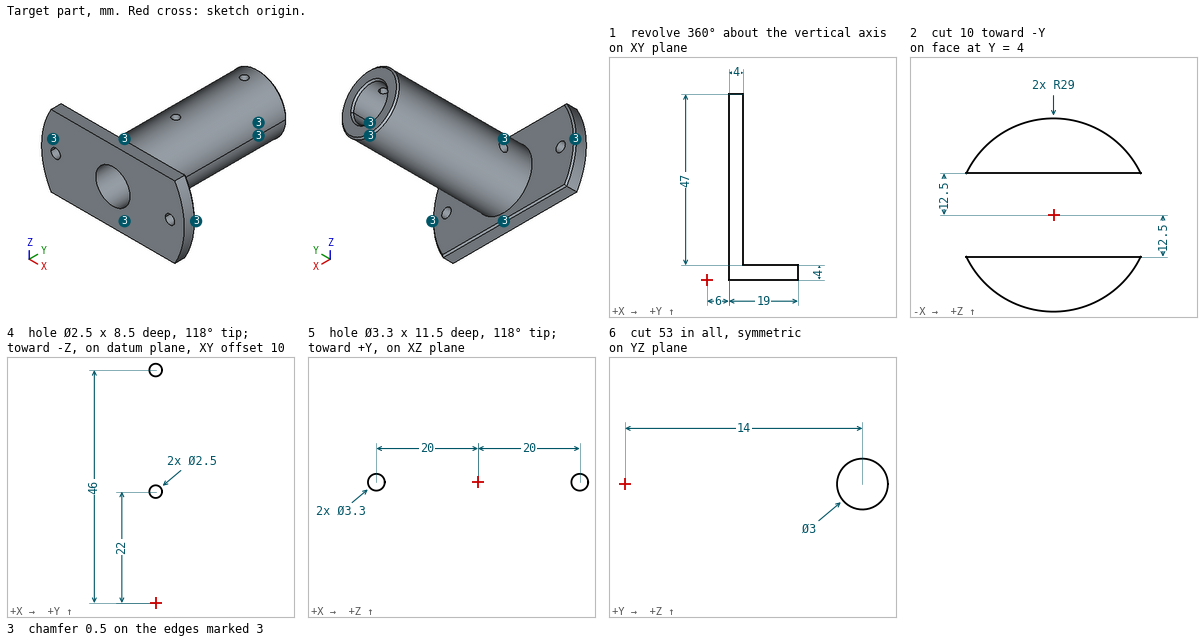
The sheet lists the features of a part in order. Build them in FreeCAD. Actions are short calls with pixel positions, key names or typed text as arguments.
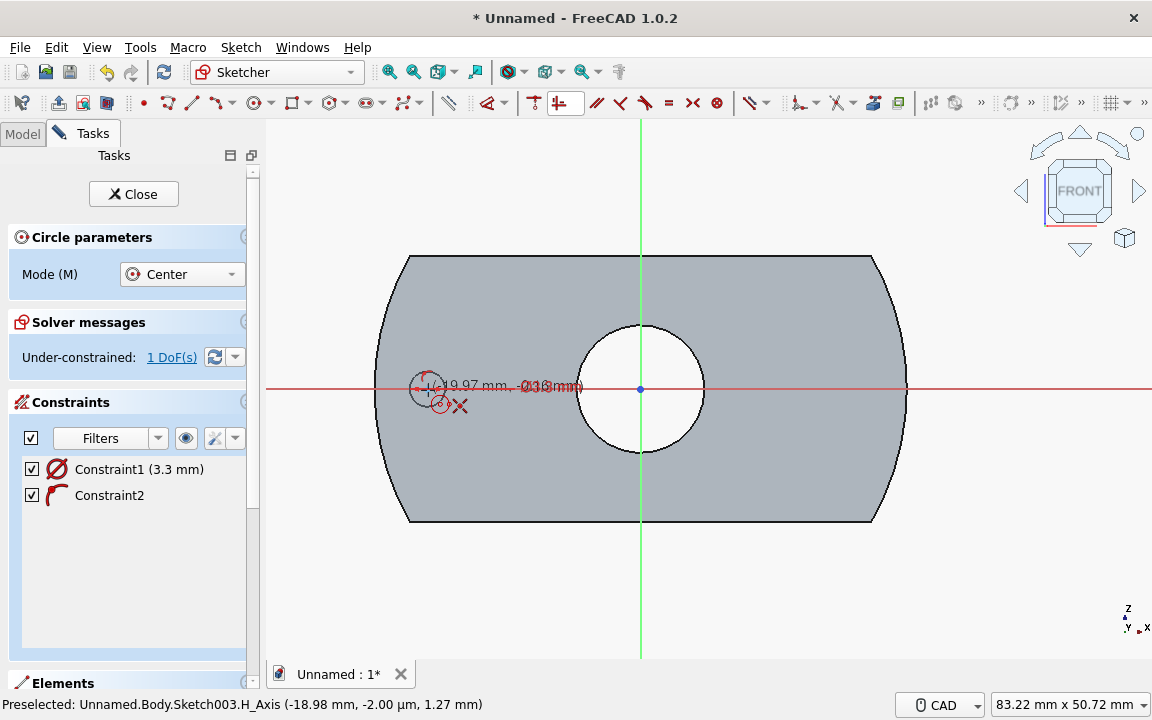
scroll(854, 389, up, 2)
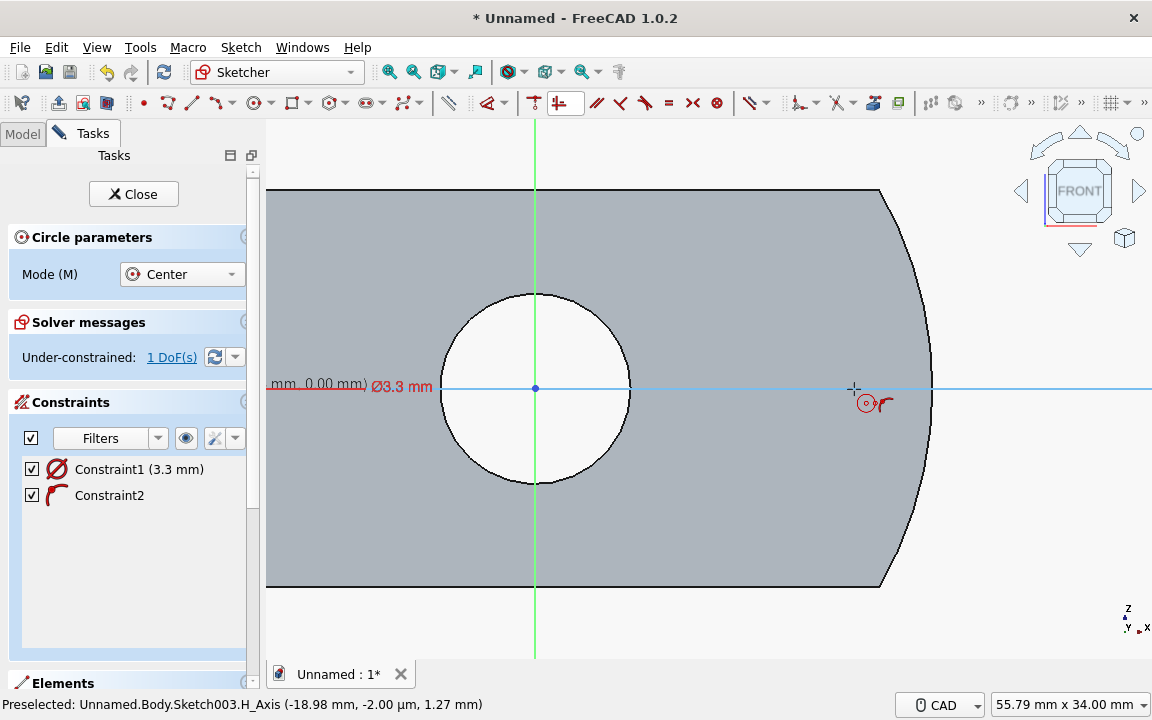
click(853, 389)
move(872, 370)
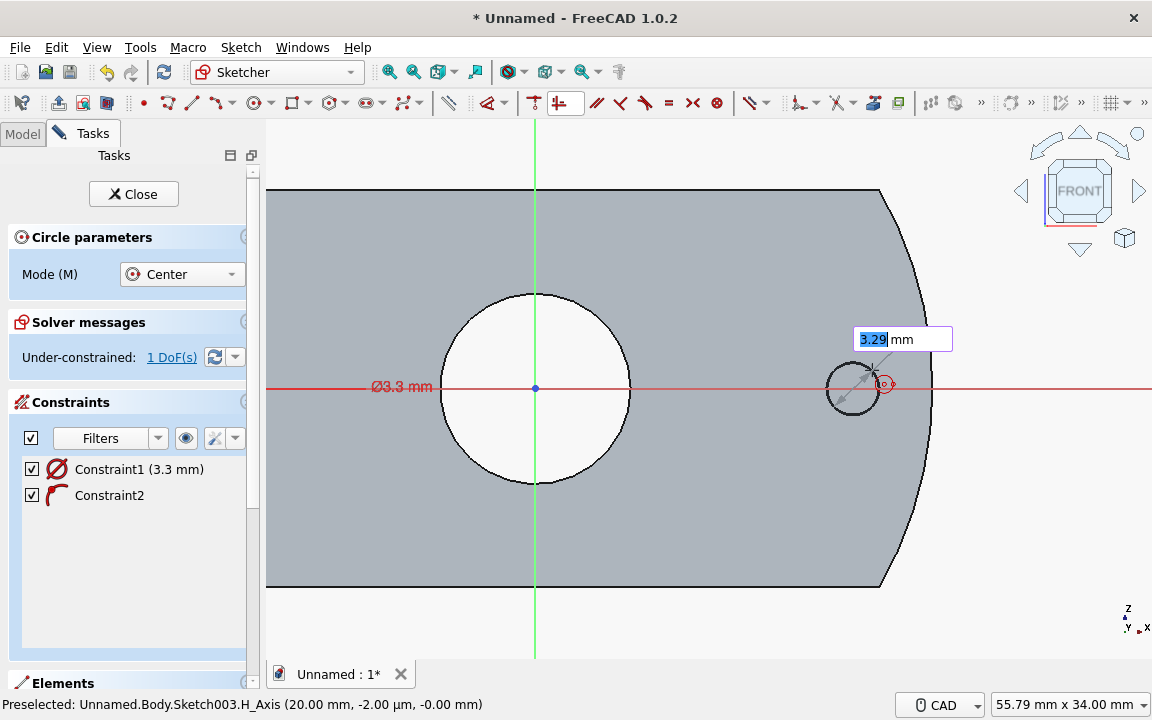
text(3.3)
key(Return)
key(Escape)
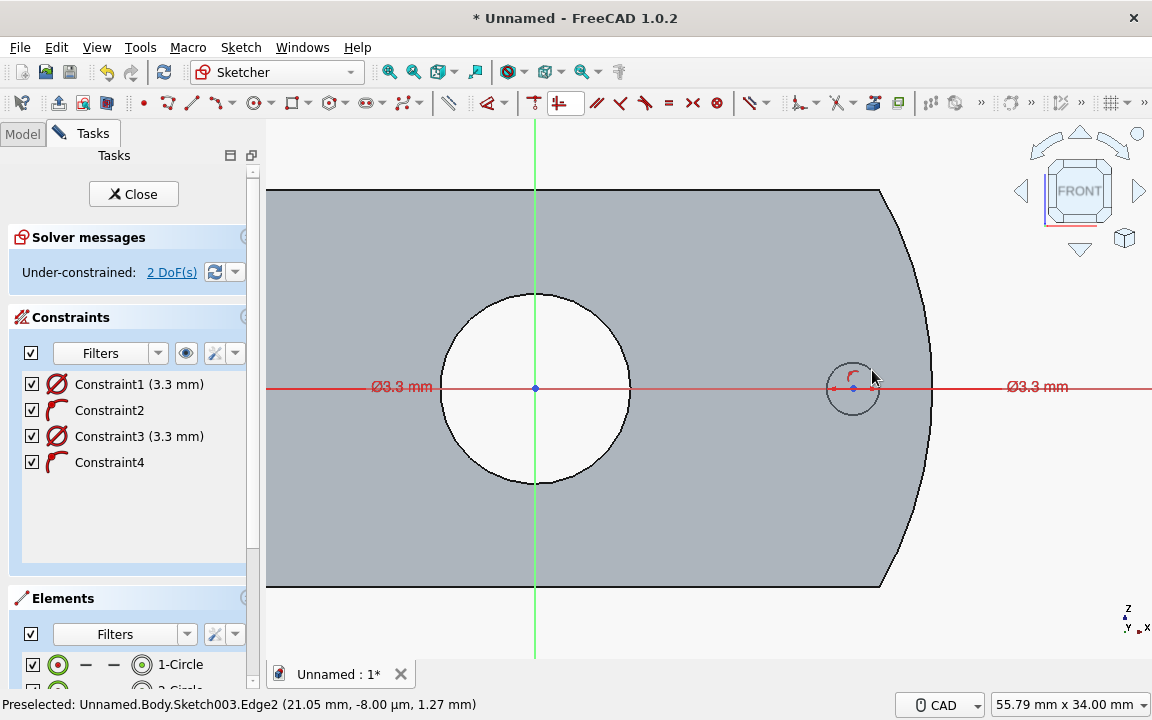
click(488, 104)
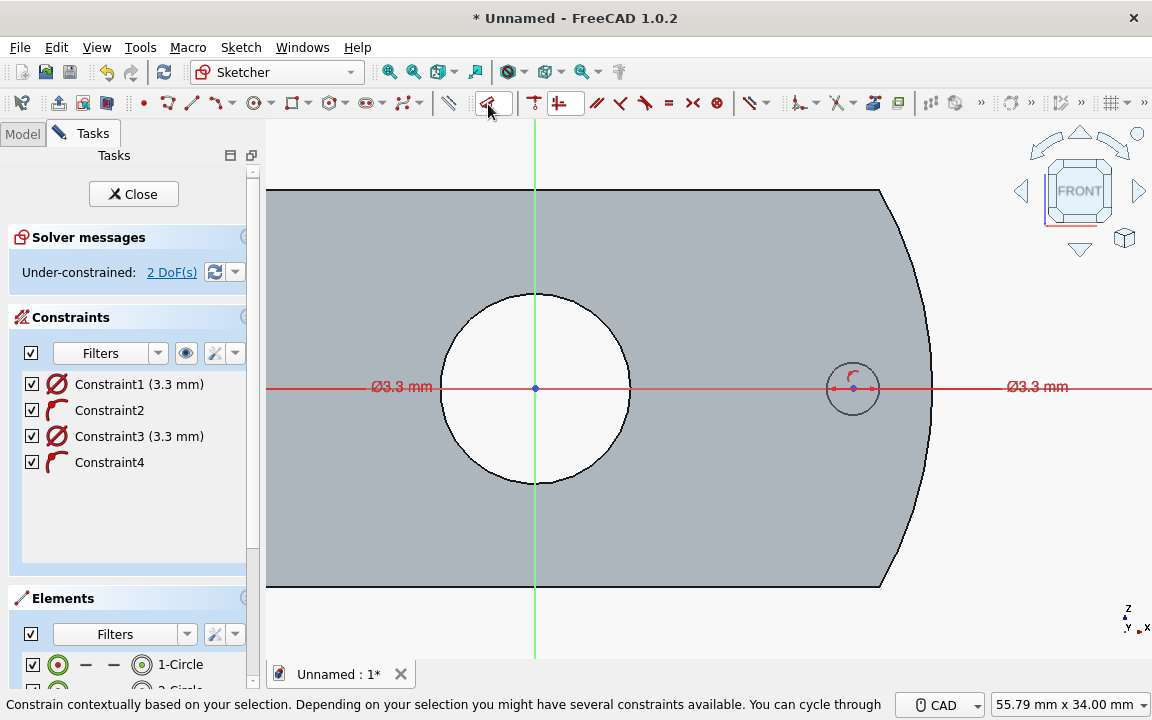
scroll(854, 389, down, 2)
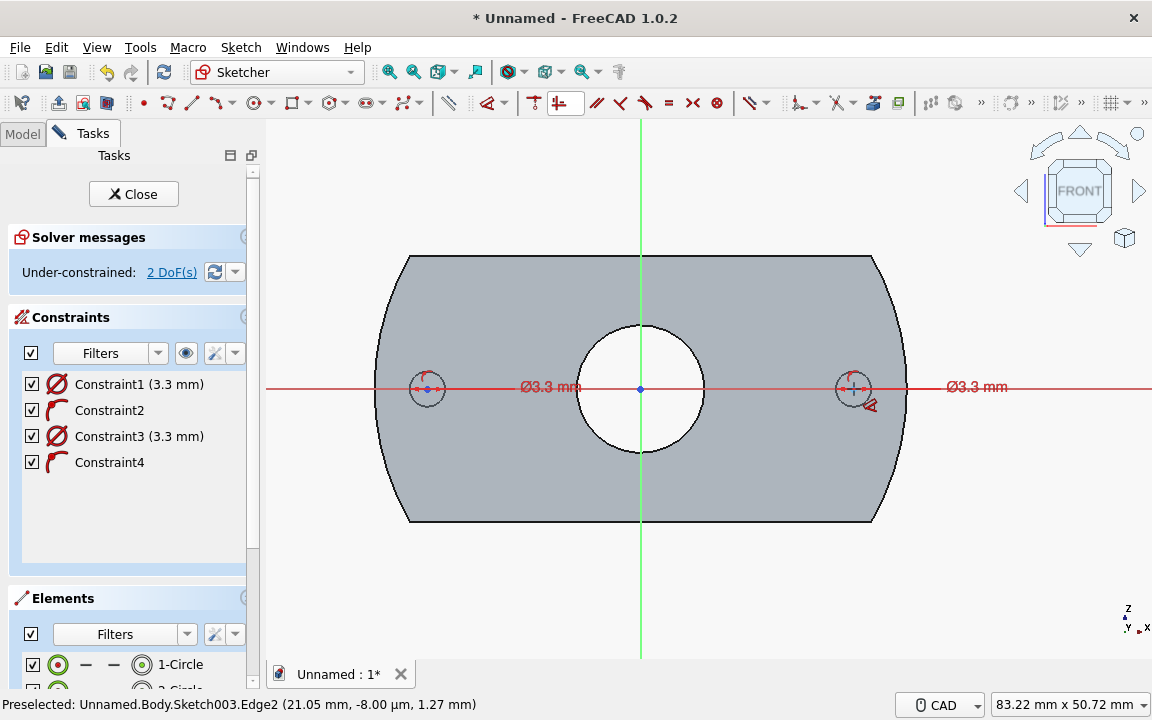
click(427, 389)
click(534, 423)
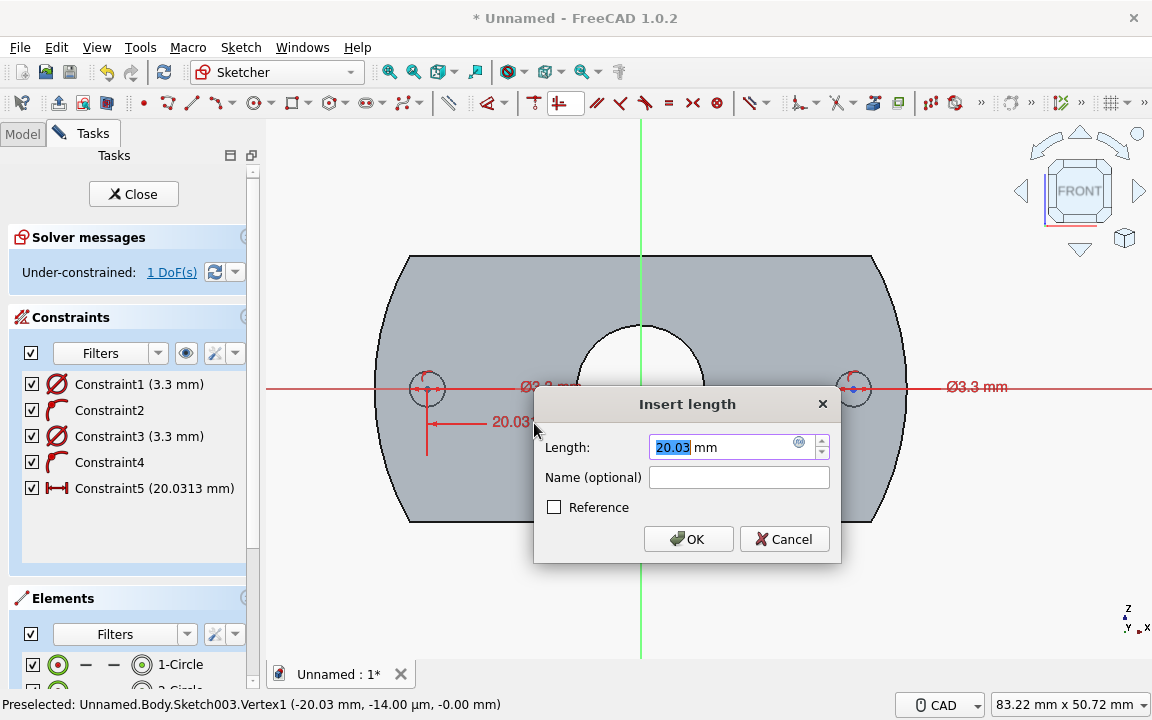
text(20)
key(Return)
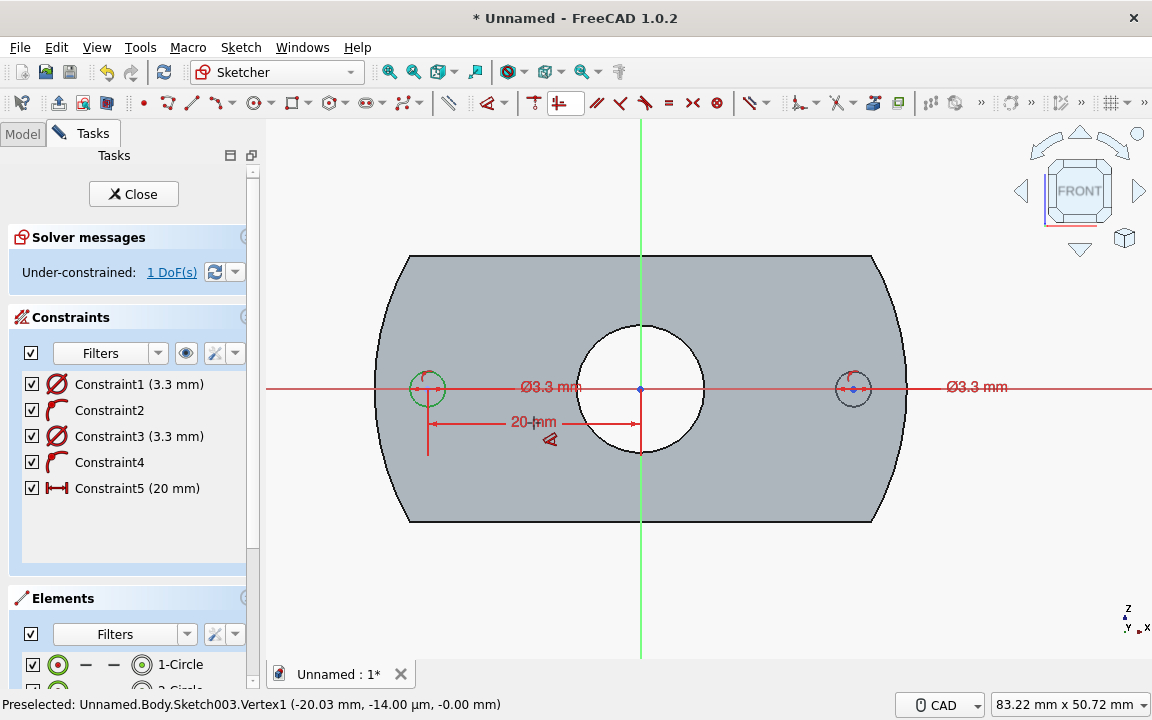
click(854, 389)
click(747, 423)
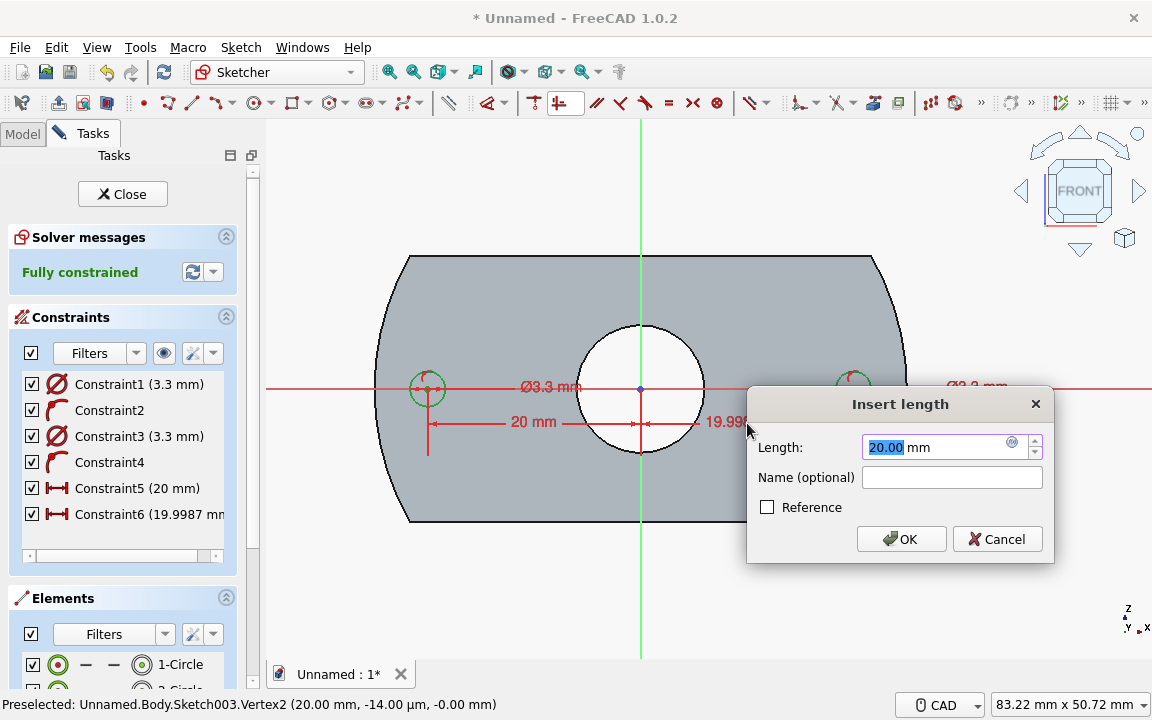
text(20)
key(Return)
key(Escape)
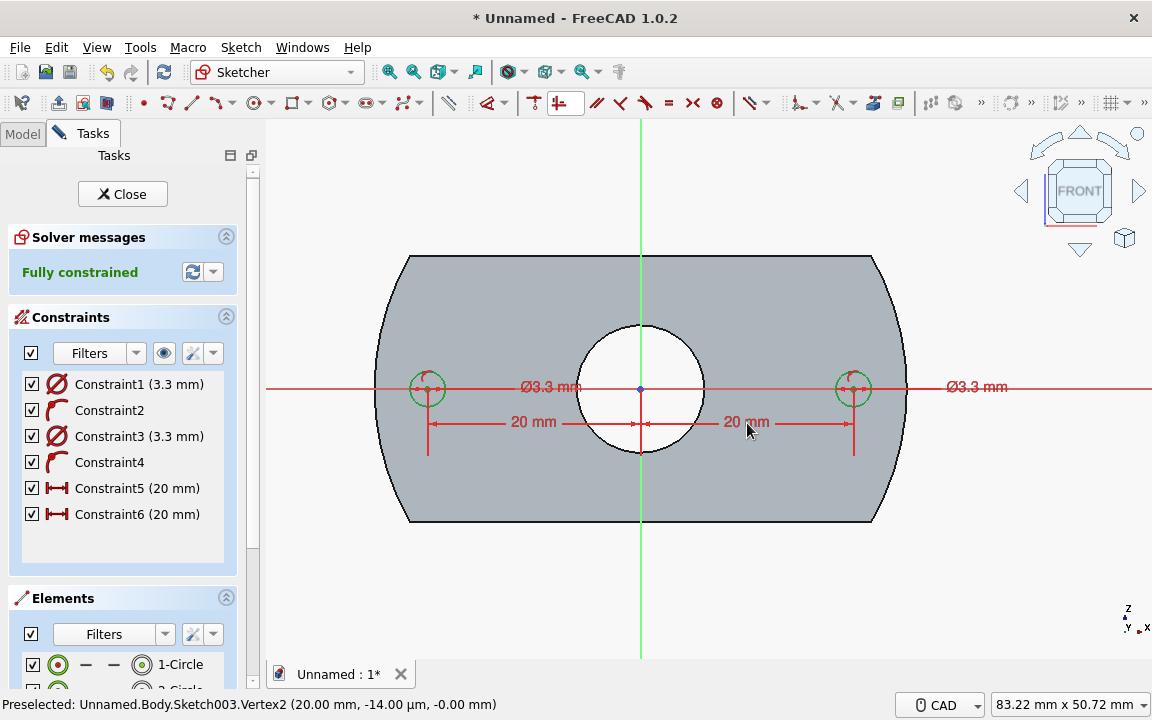
click(123, 194)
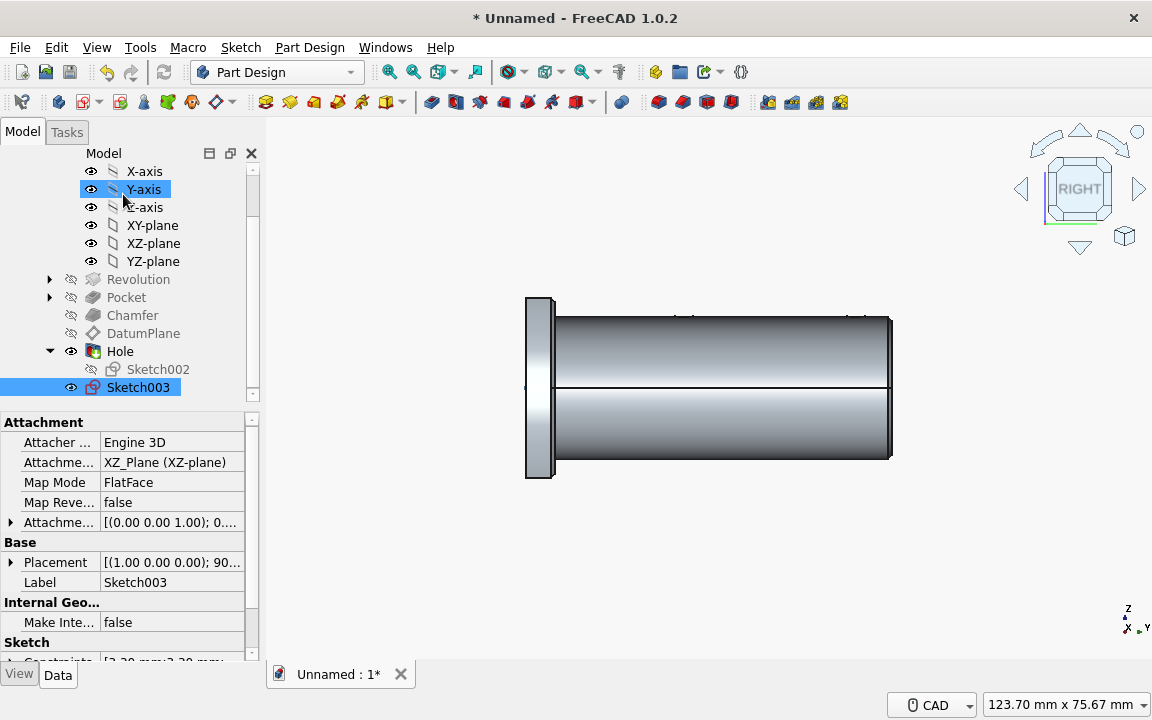
click(456, 102)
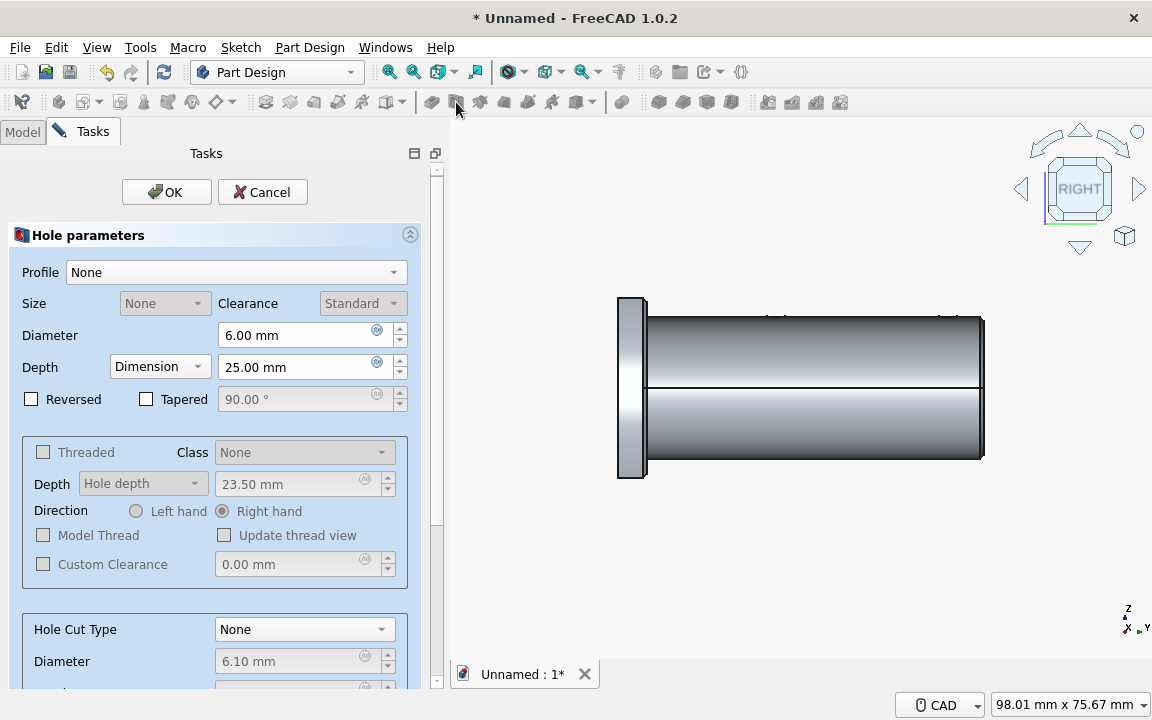
triple_click(305, 335)